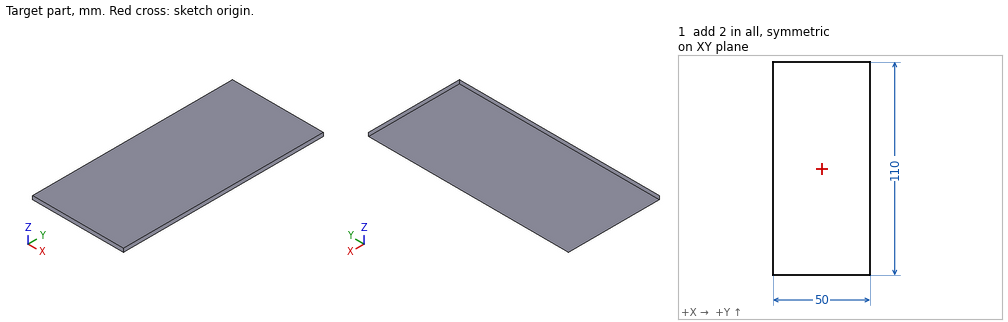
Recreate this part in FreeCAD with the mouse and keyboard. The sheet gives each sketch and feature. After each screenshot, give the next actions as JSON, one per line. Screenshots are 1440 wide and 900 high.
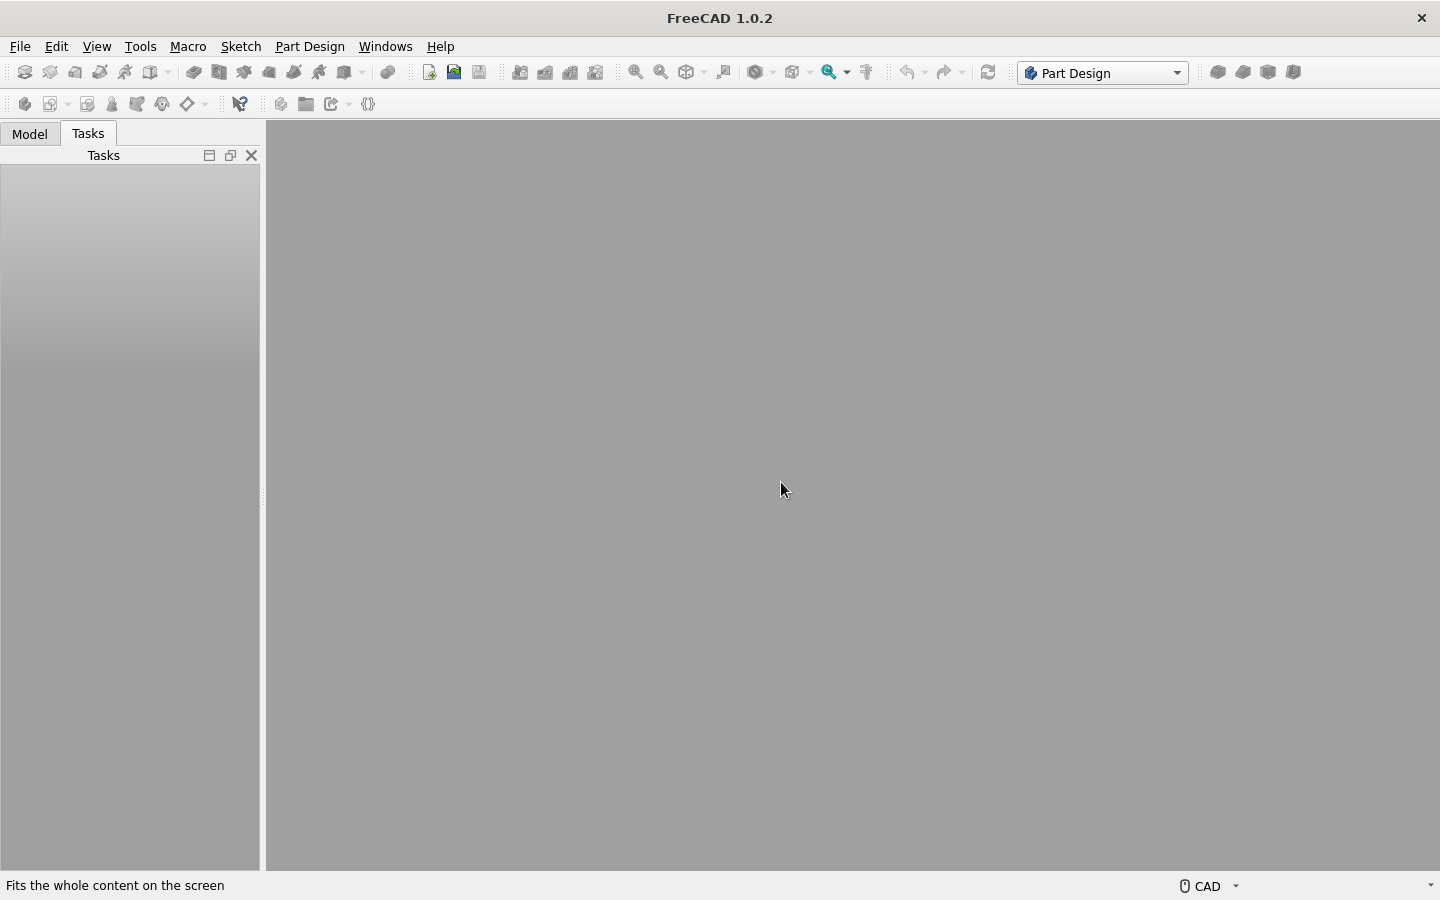
{"action": "left_click", "coordinate": [429, 72]}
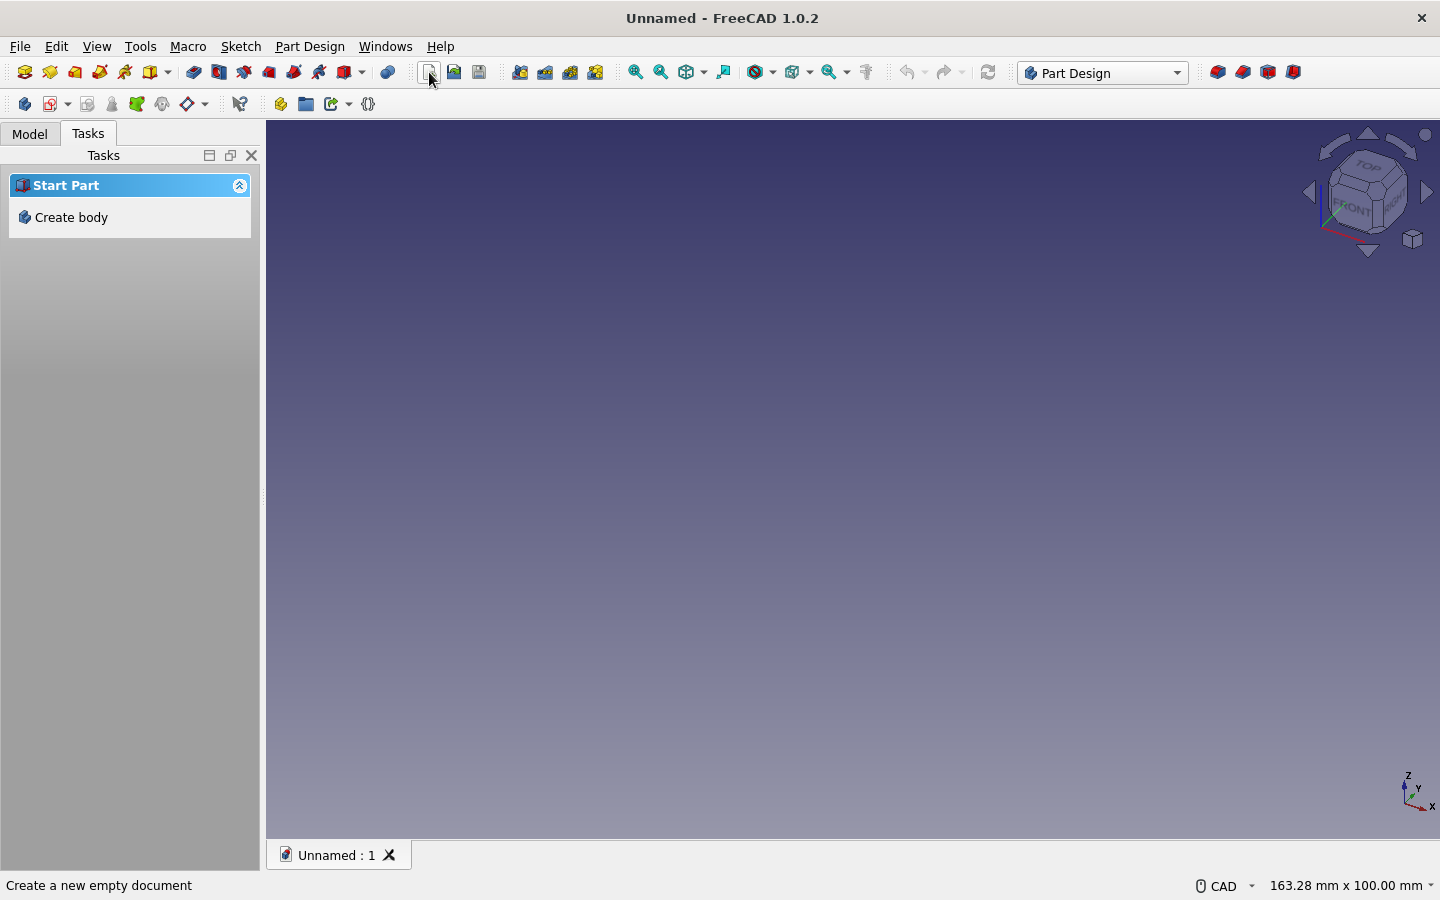
{"action": "left_click", "coordinate": [50, 104]}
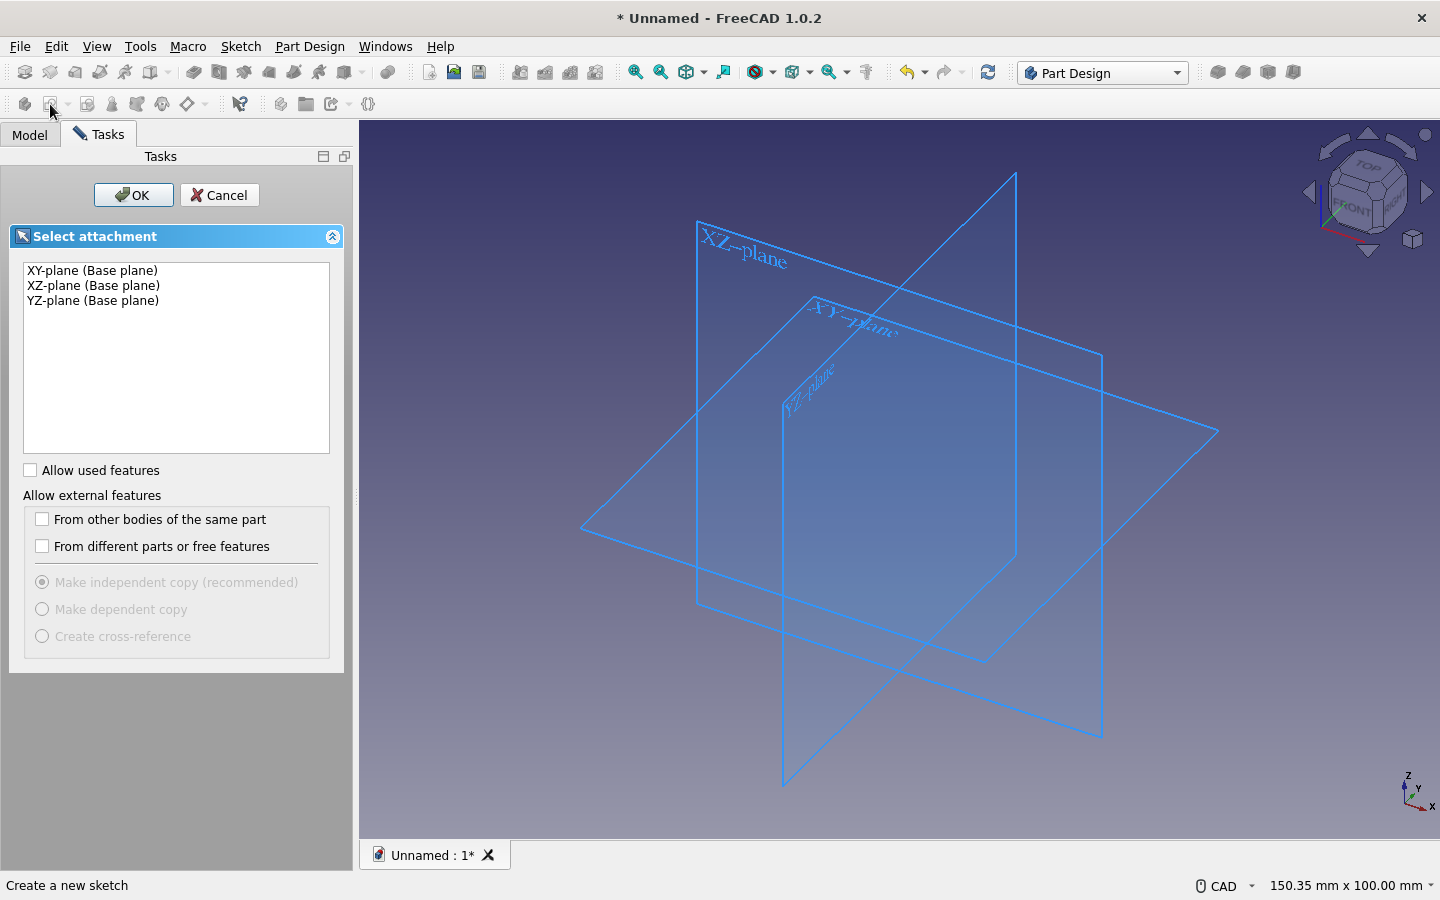
{"action": "left_click", "coordinate": [84, 270]}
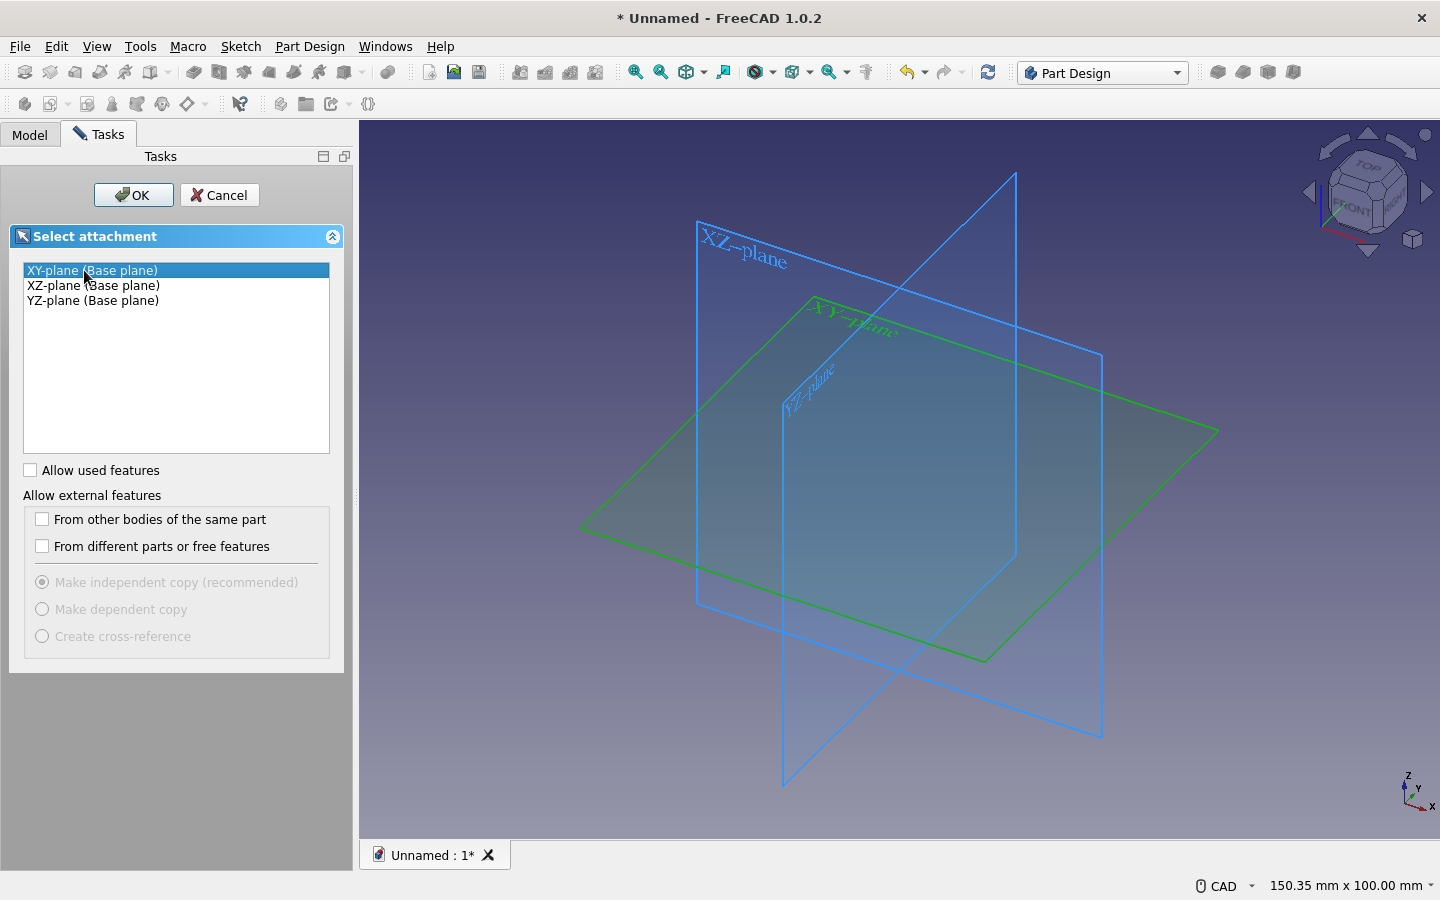
{"action": "left_click", "coordinate": [134, 195]}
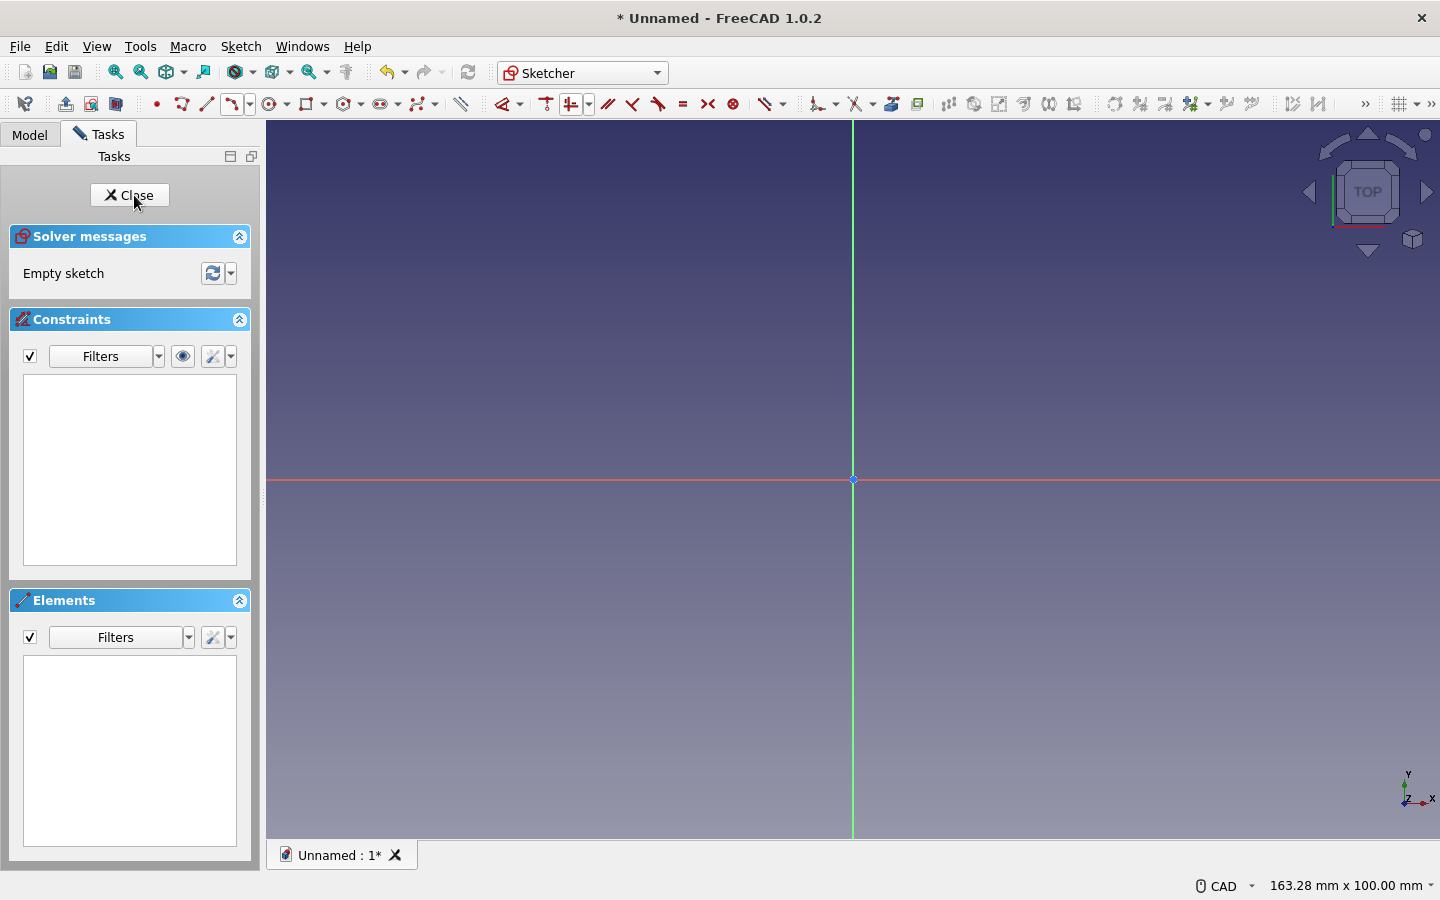
{"action": "scroll", "coordinate": [701, 479], "scroll_direction": "down", "scroll_amount": 3}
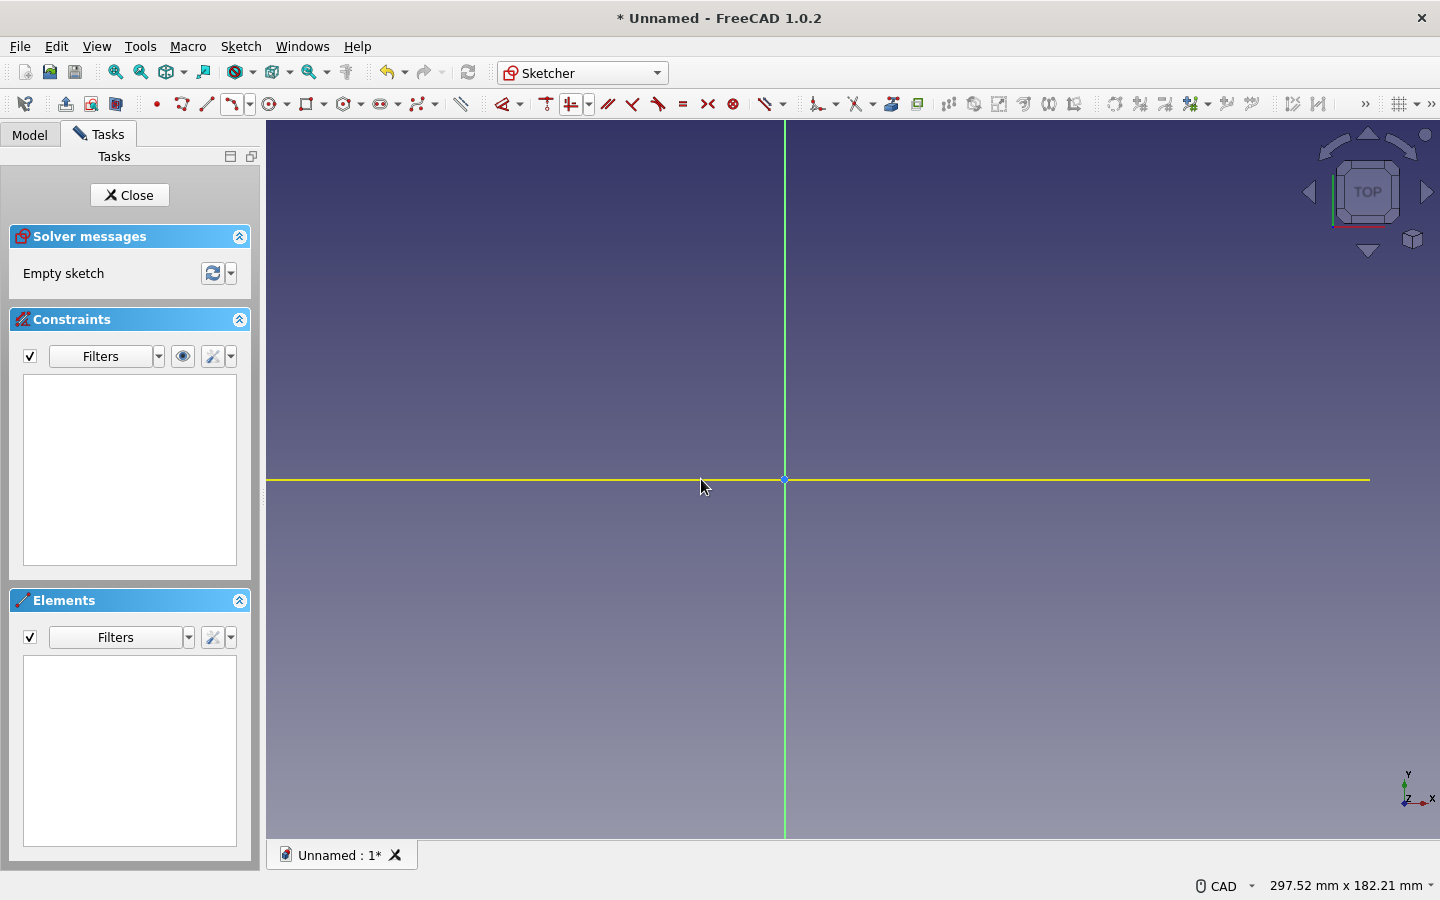
{"action": "left_click", "coordinate": [324, 104]}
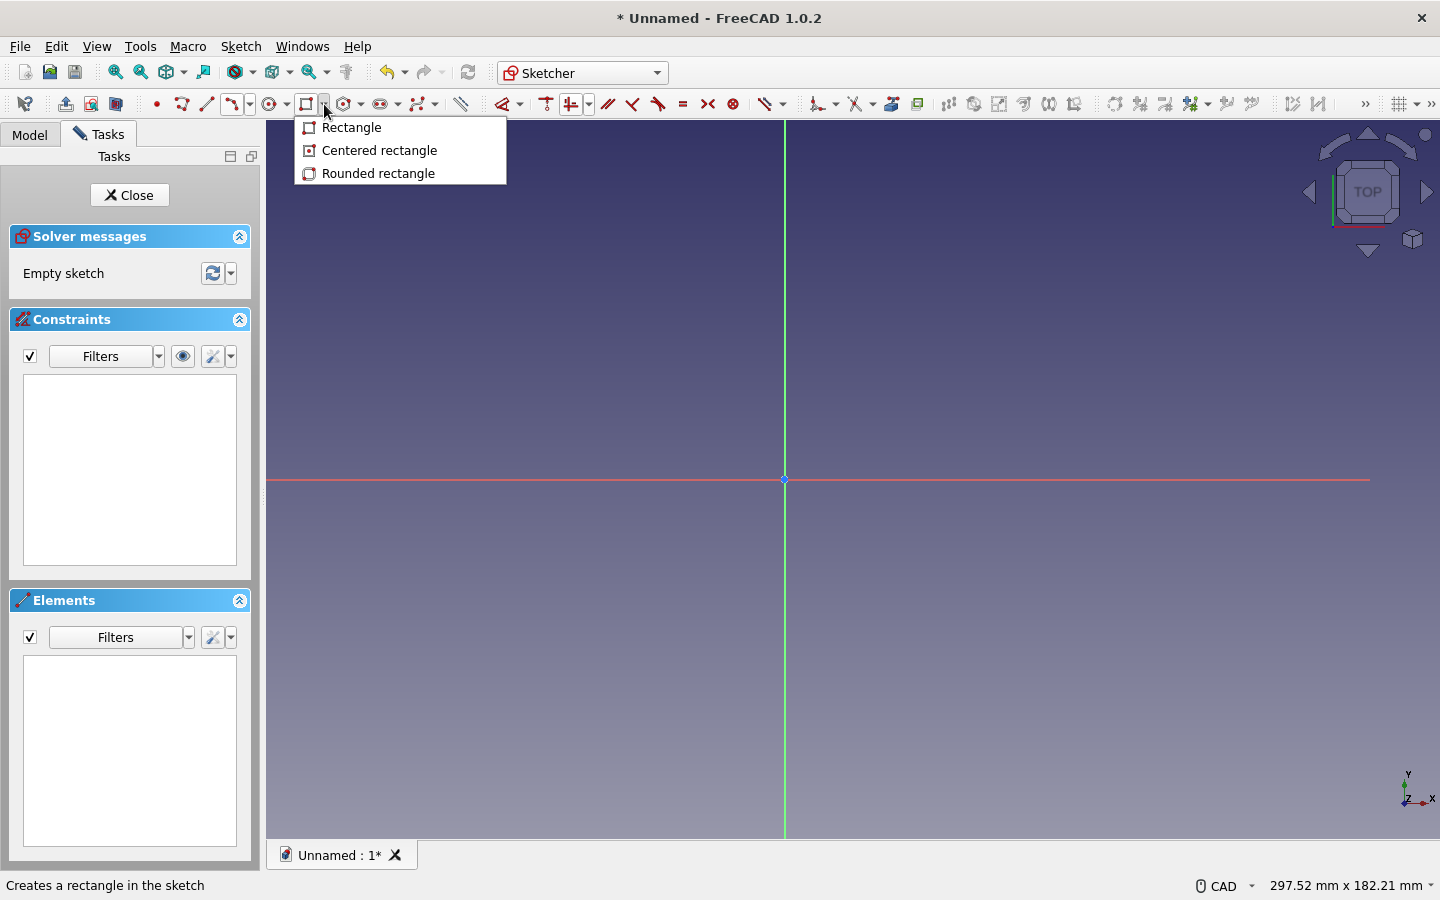
{"action": "left_click", "coordinate": [400, 150]}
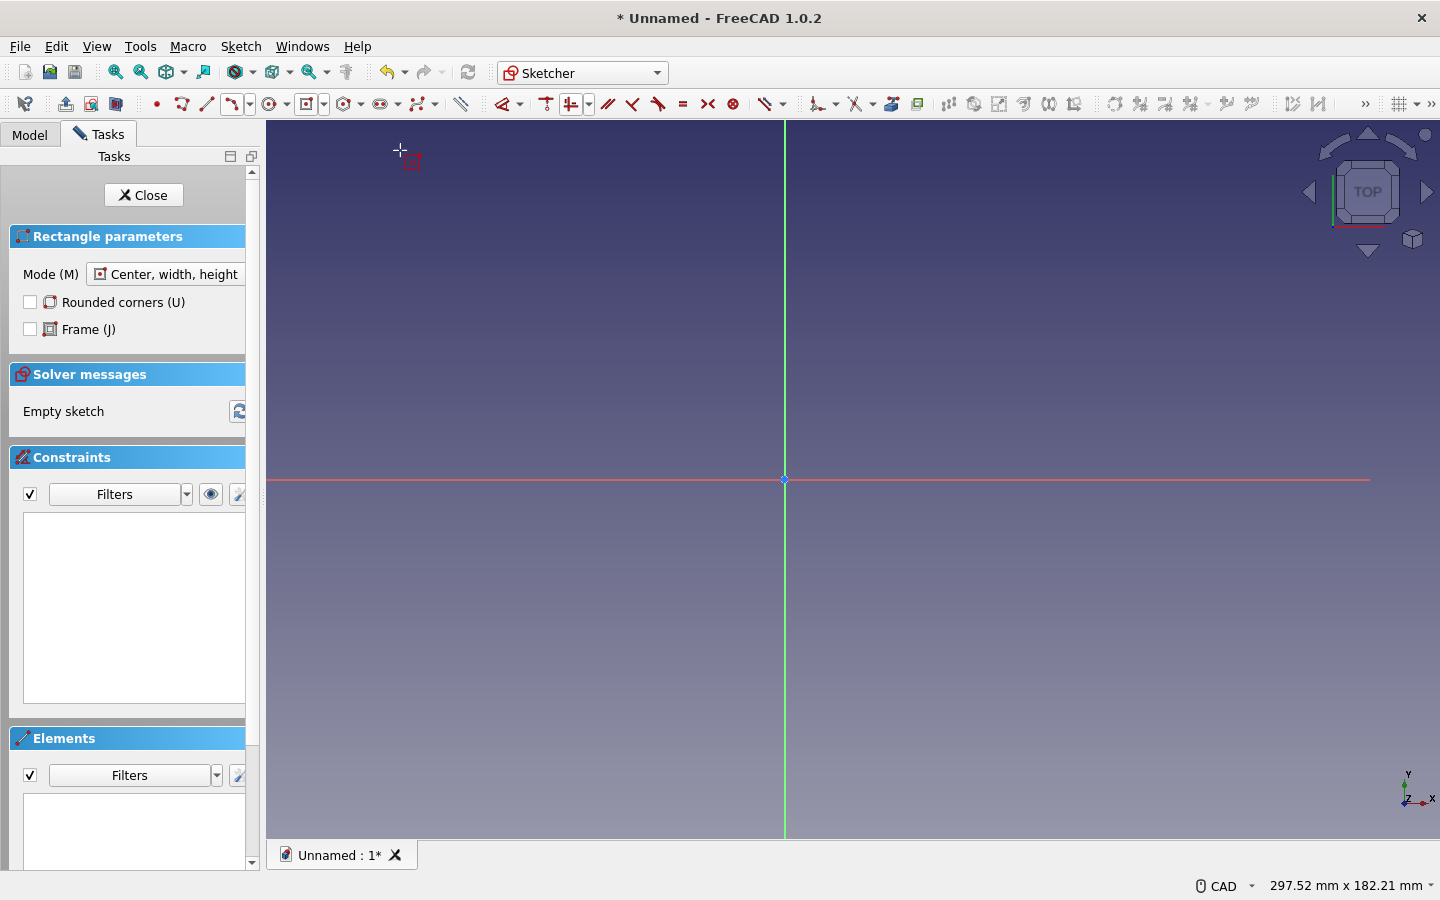
{"action": "left_click", "coordinate": [785, 480]}
{"action": "left_click", "coordinate": [883, 262]}
{"action": "key", "text": "Escape"}